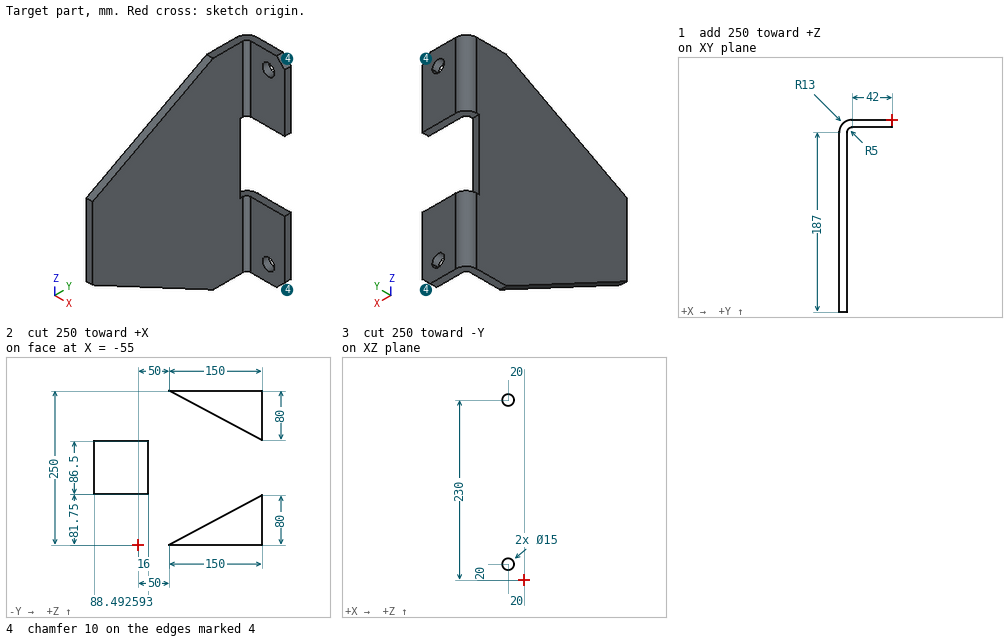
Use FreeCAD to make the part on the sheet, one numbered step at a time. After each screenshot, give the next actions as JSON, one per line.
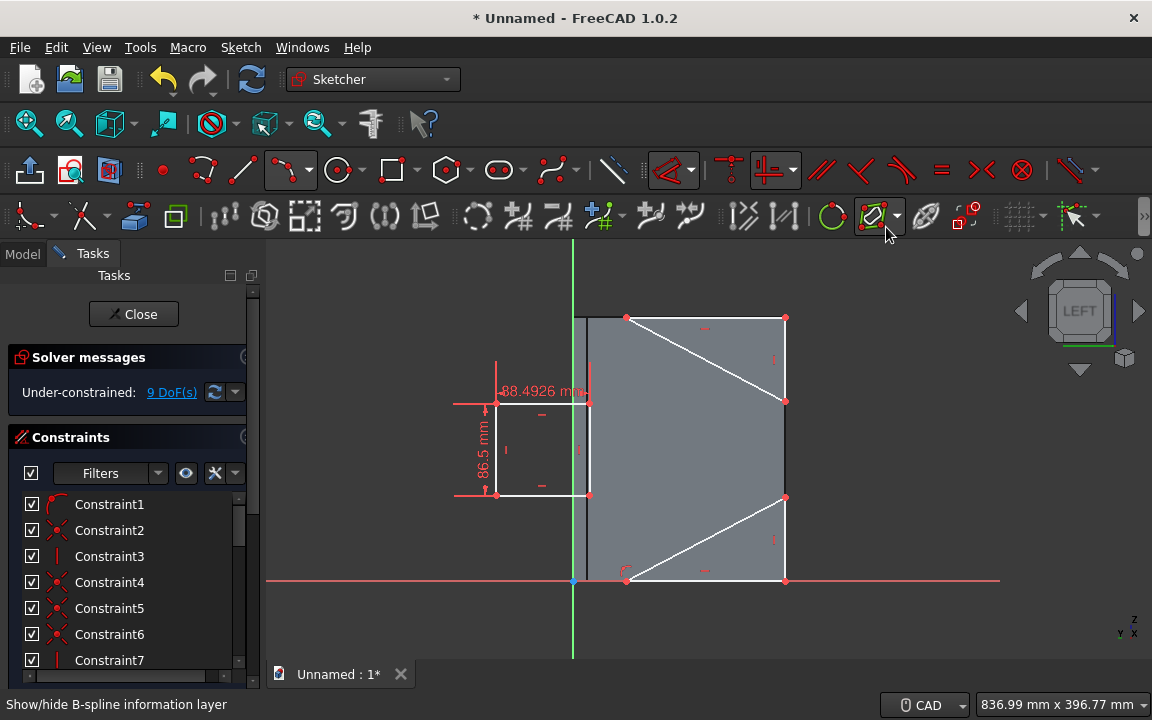
{"action": "left_click", "coordinate": [785, 556]}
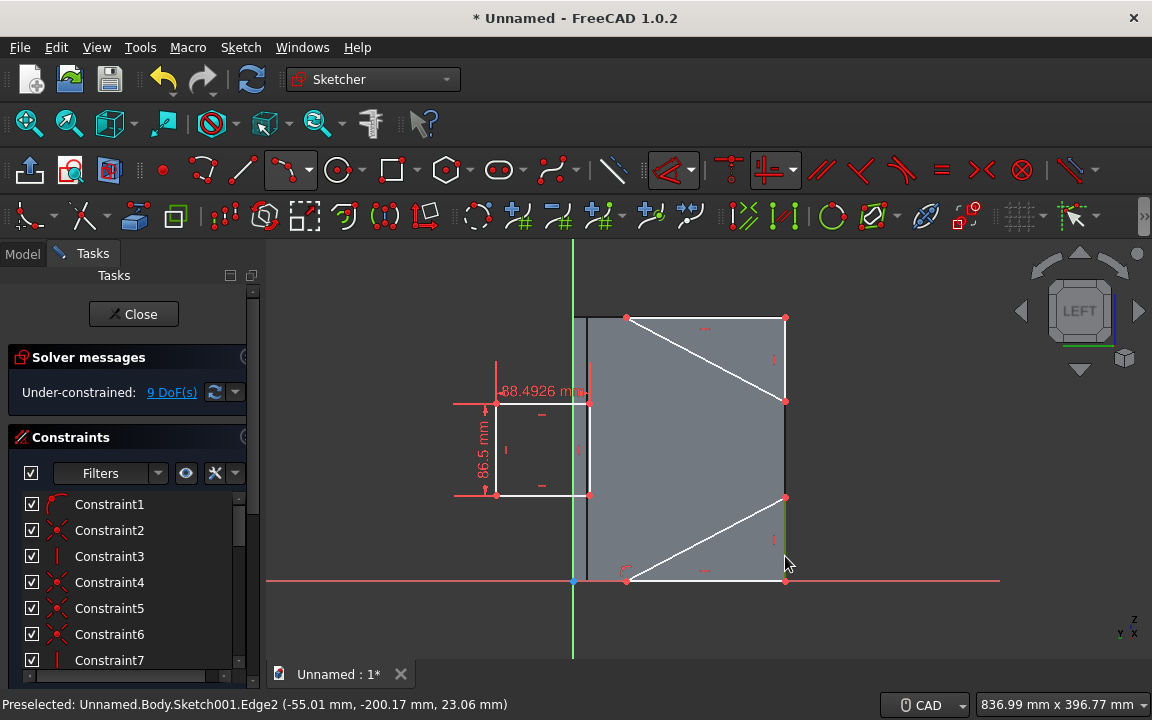
{"action": "left_click", "coordinate": [694, 170]}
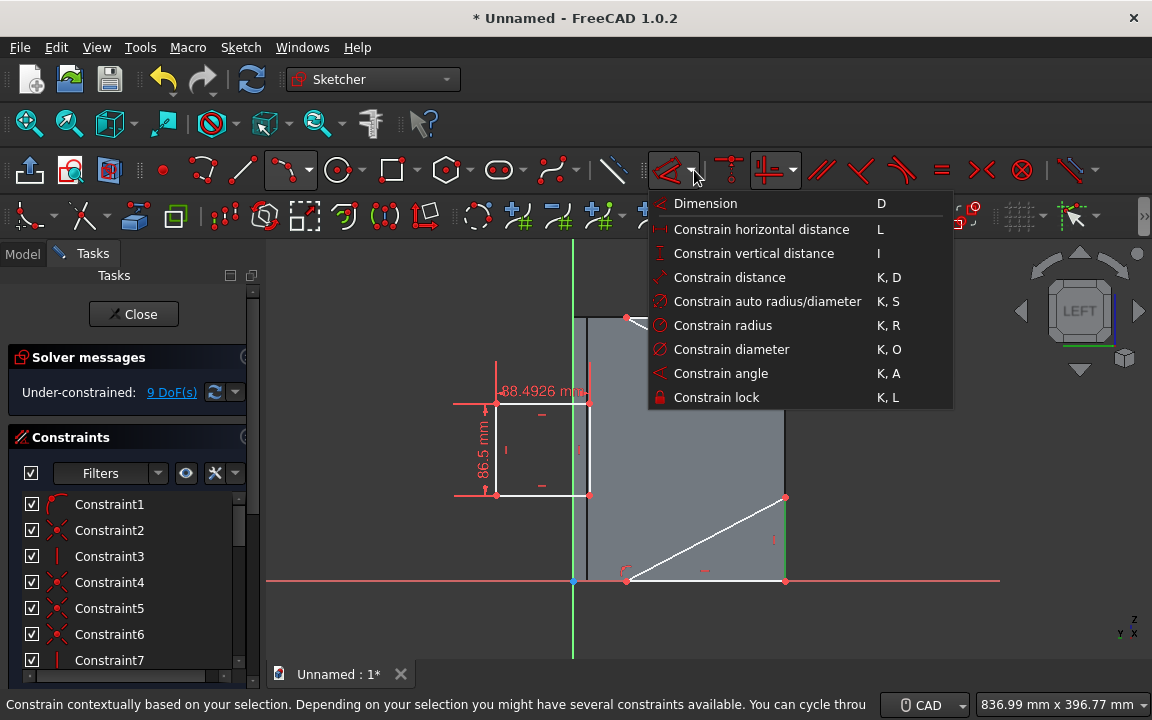
{"action": "left_click", "coordinate": [801, 253]}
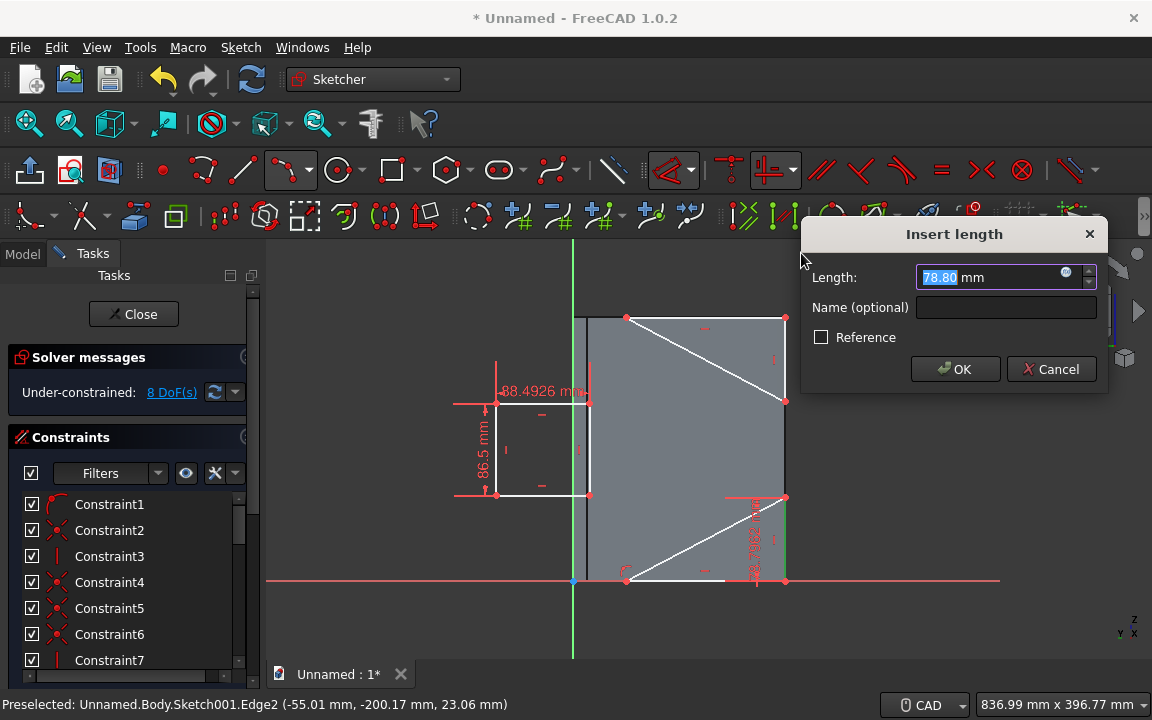
{"action": "type", "text": "80"}
{"action": "key", "text": "Return"}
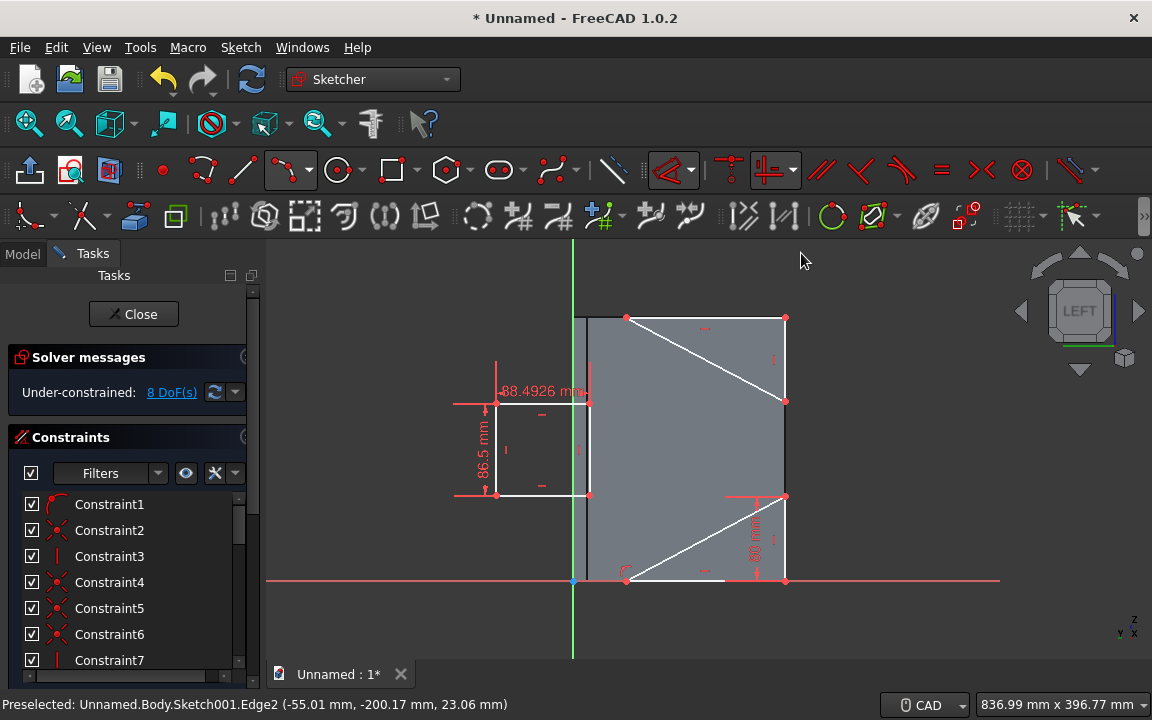
{"action": "left_click", "coordinate": [785, 377]}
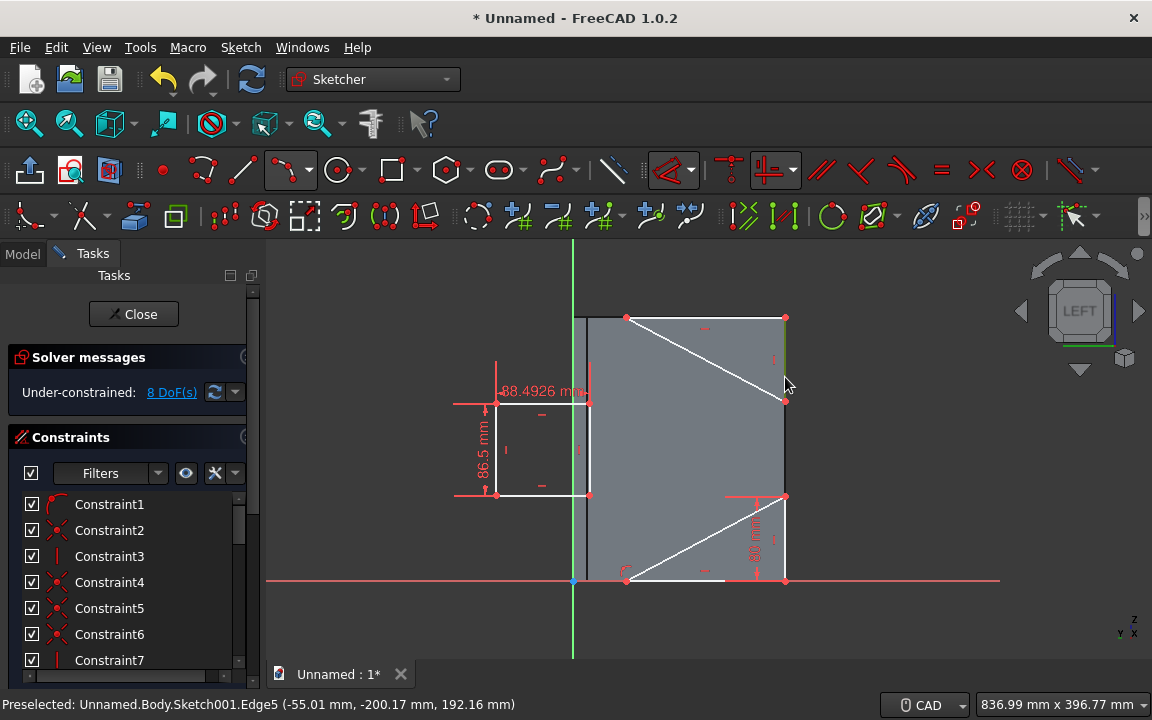
{"action": "key", "text": "i"}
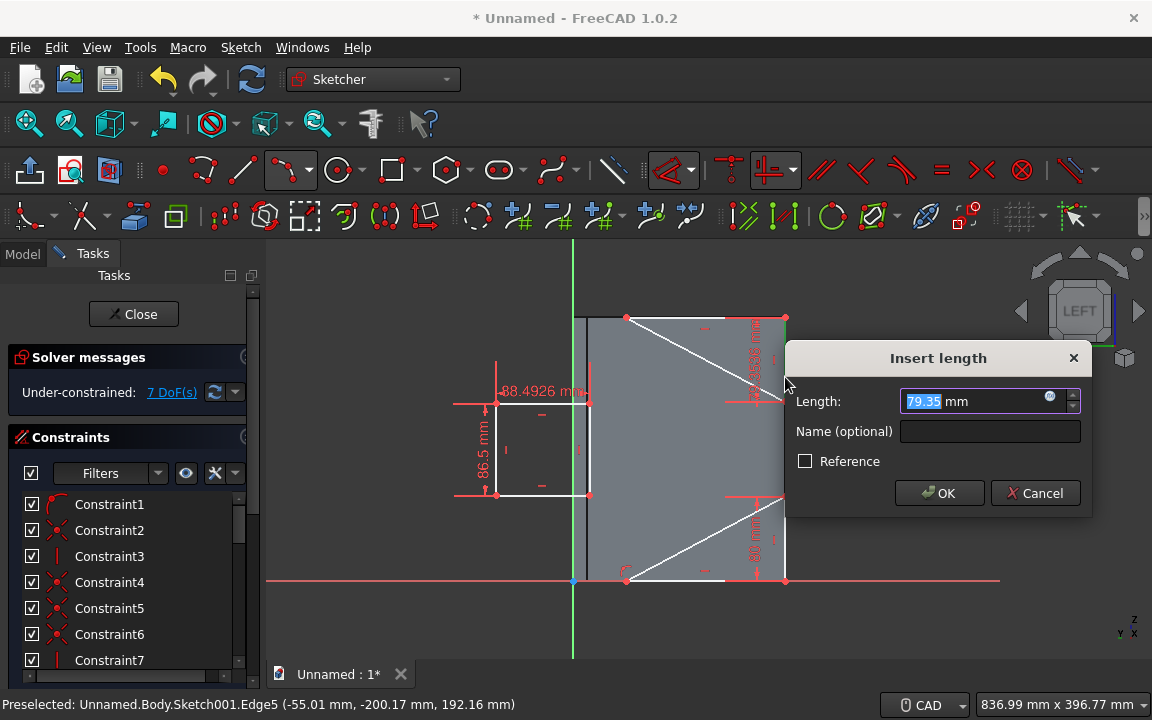
{"action": "type", "text": "80"}
{"action": "key", "text": "Return"}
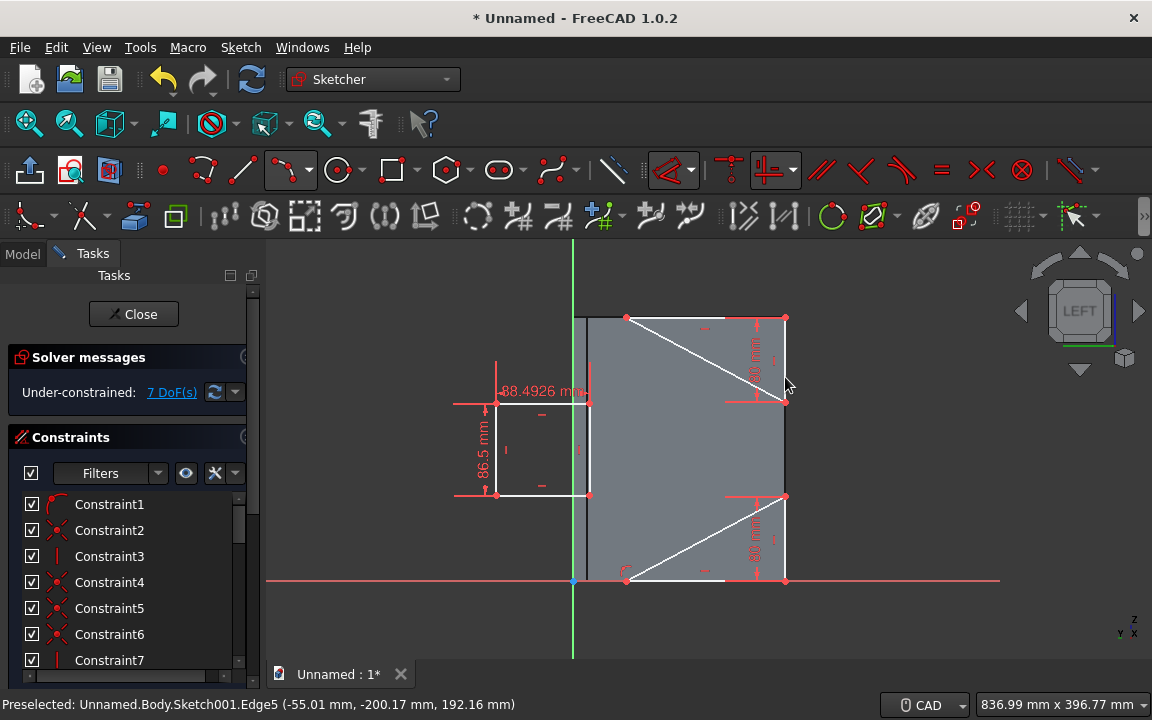
{"action": "left_click", "coordinate": [674, 581]}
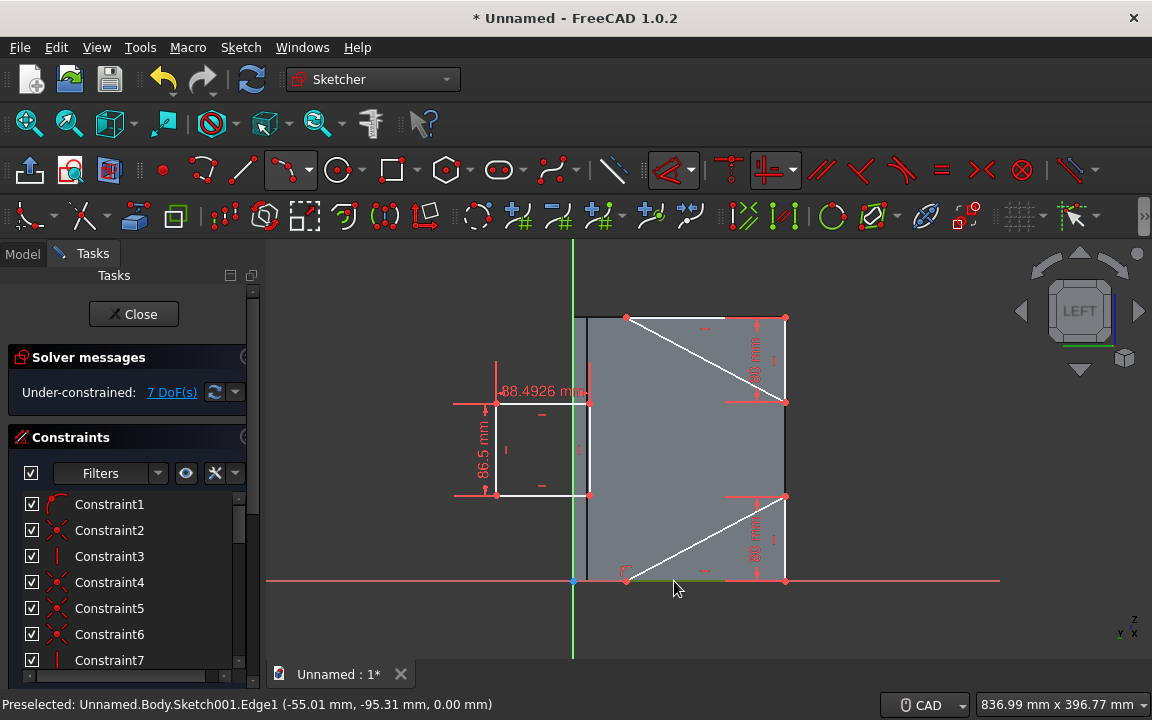
{"action": "key", "text": "l"}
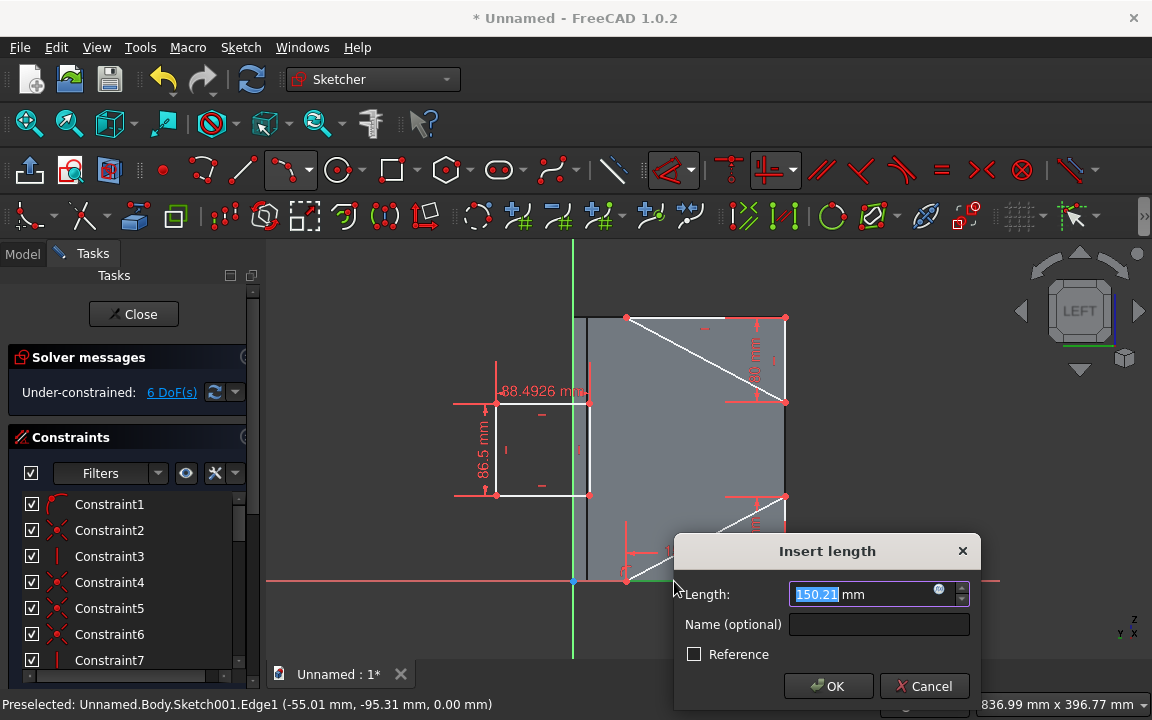
{"action": "type", "text": "150"}
{"action": "key", "text": "Return"}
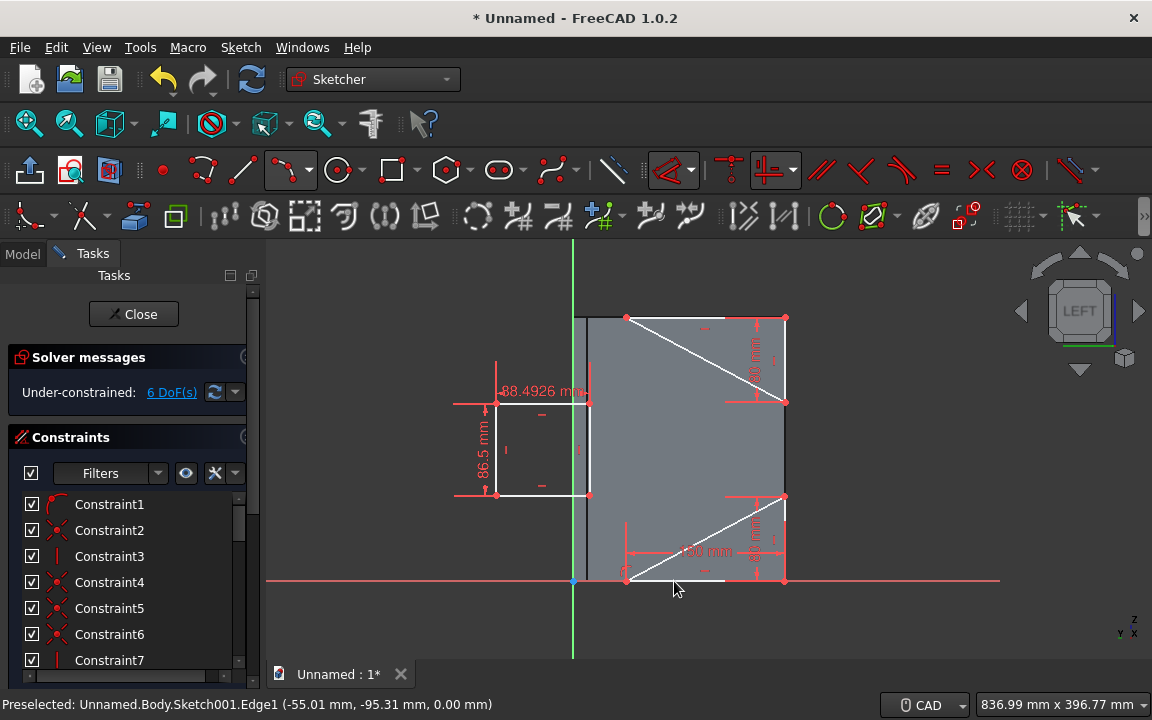
{"action": "left_click", "coordinate": [737, 318]}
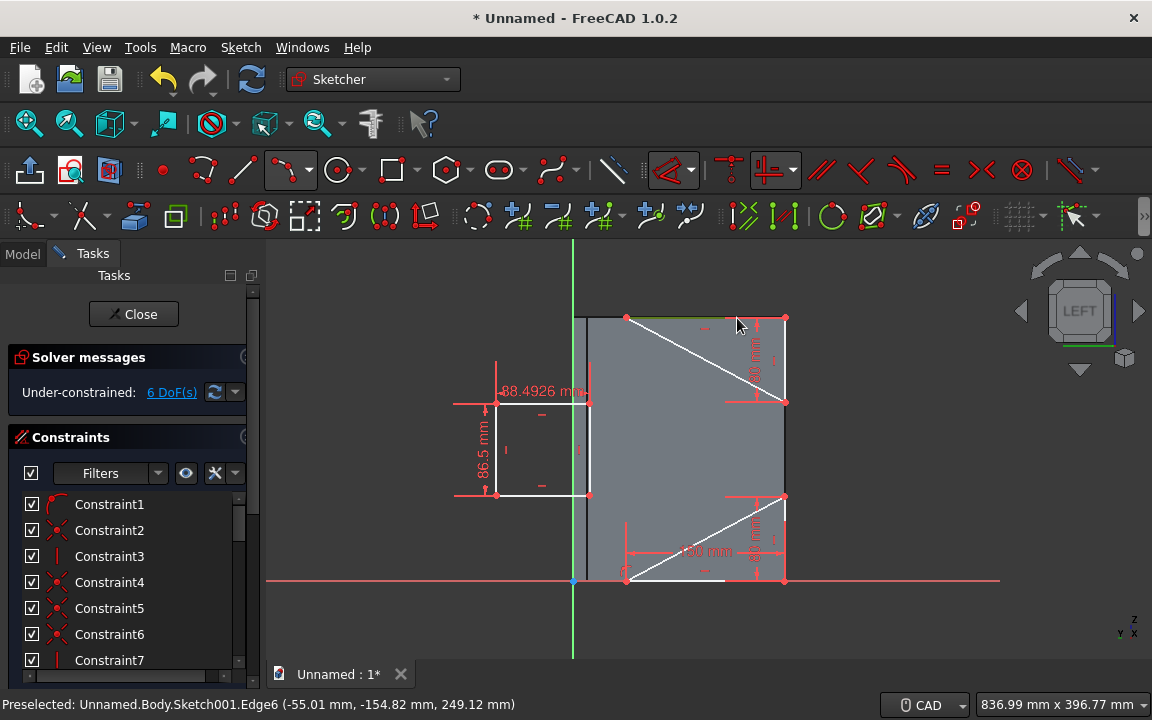
{"action": "left_click", "coordinate": [694, 170]}